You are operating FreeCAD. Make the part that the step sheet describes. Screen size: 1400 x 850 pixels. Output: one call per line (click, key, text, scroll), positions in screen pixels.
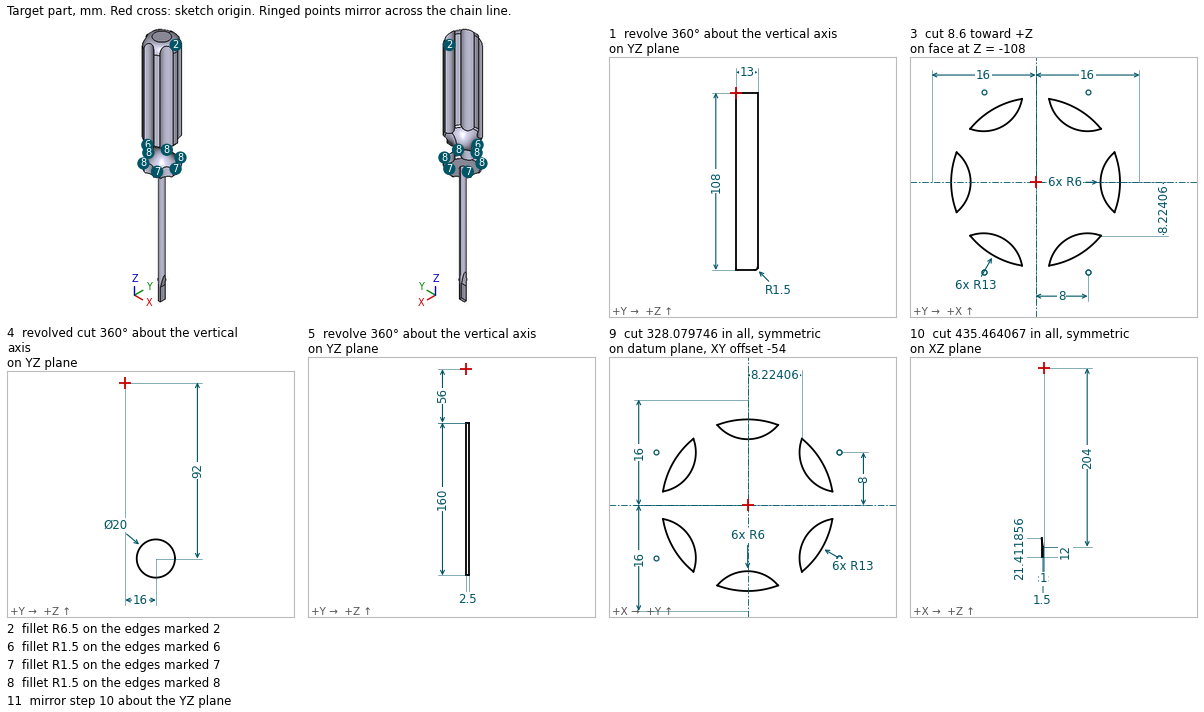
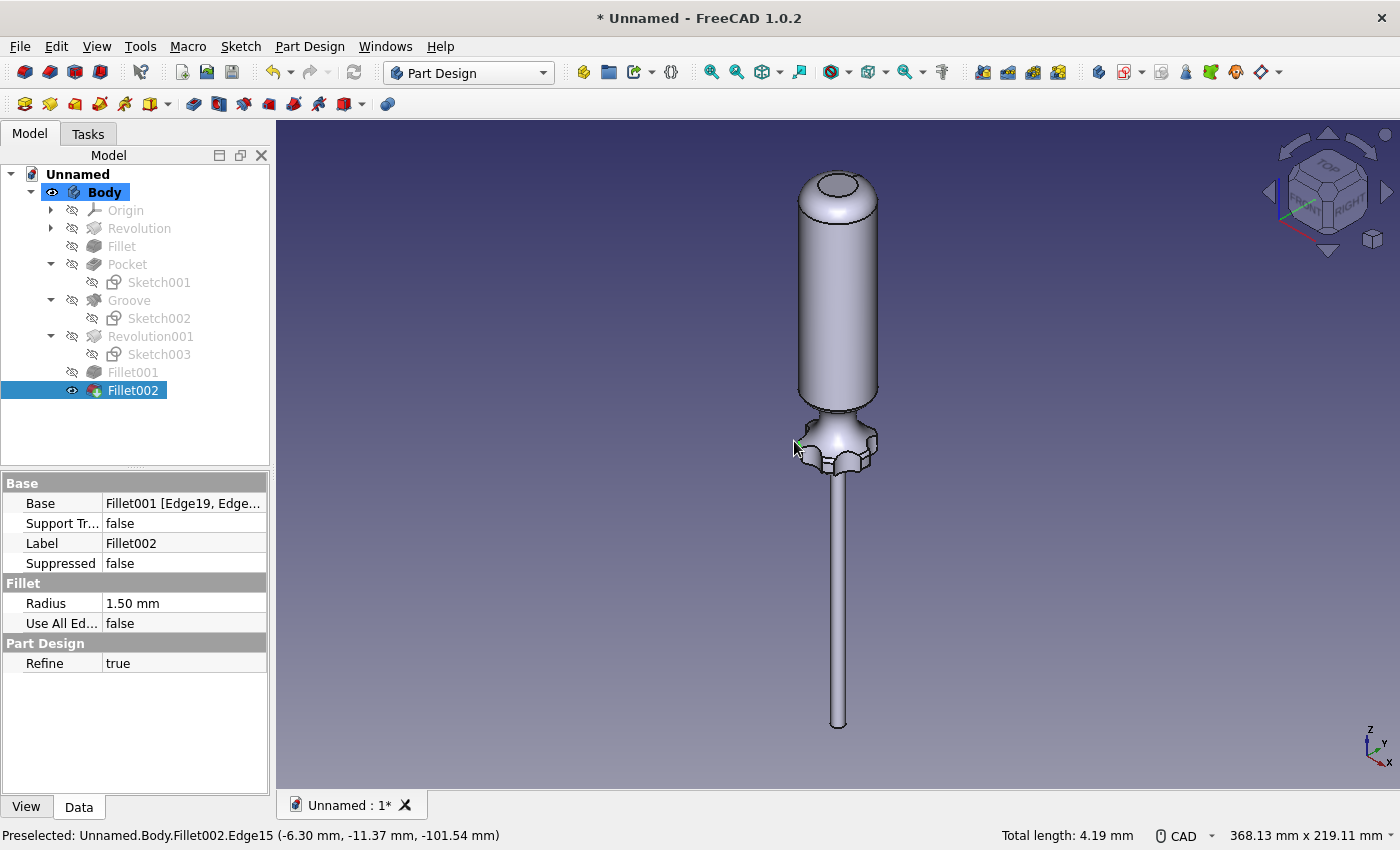
scroll(876, 431, up, 6)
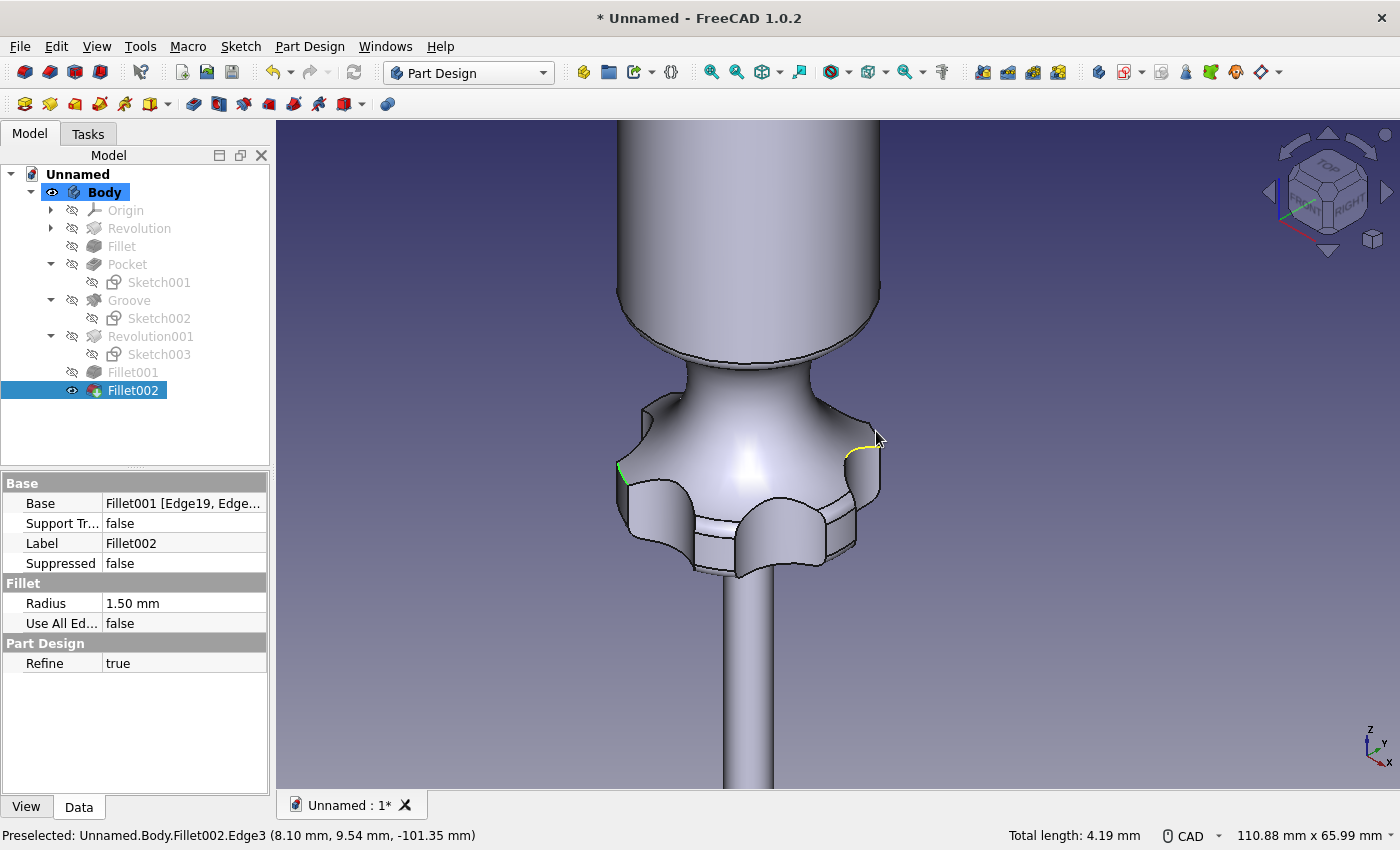
key(v)
key(f)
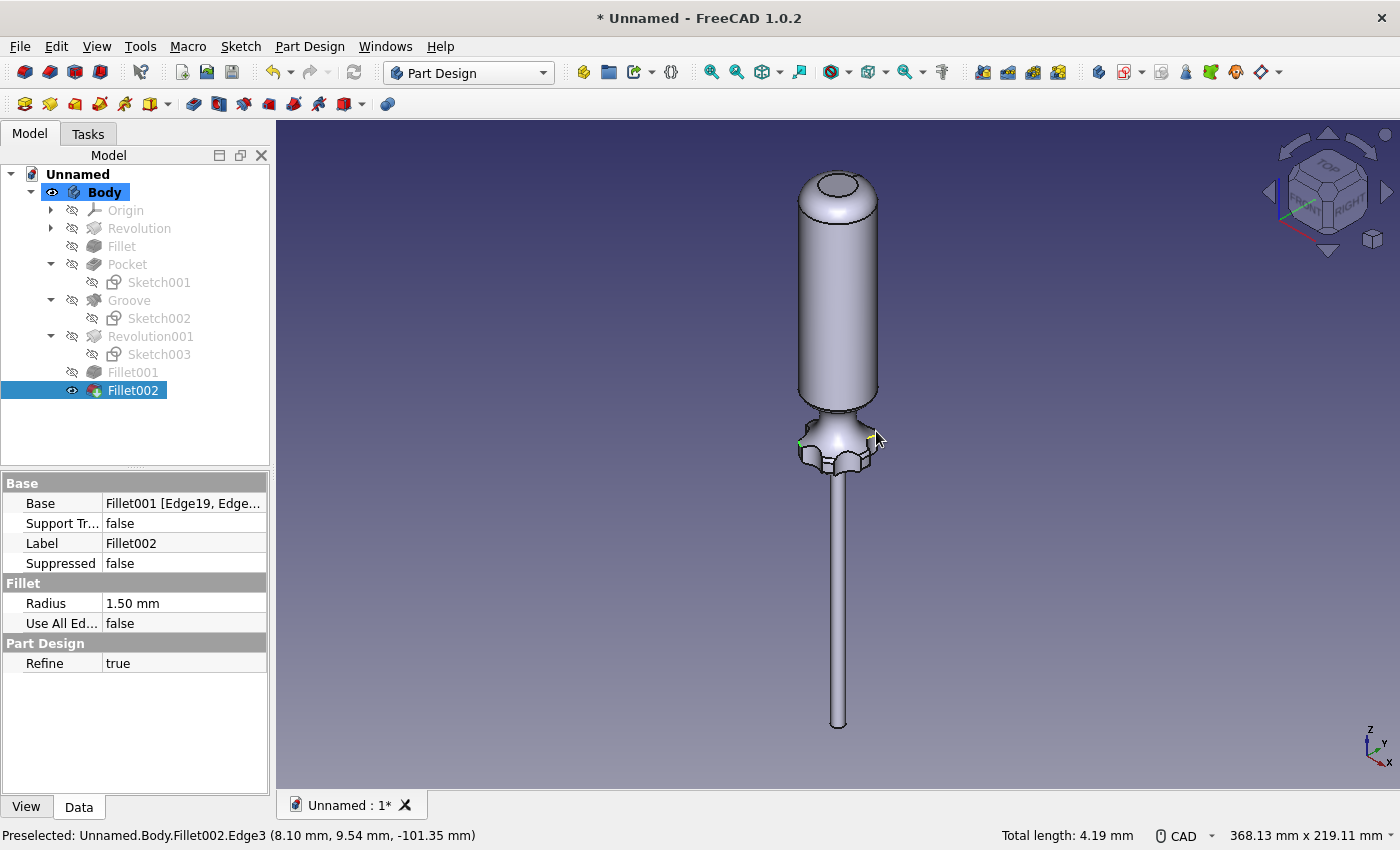
key(2)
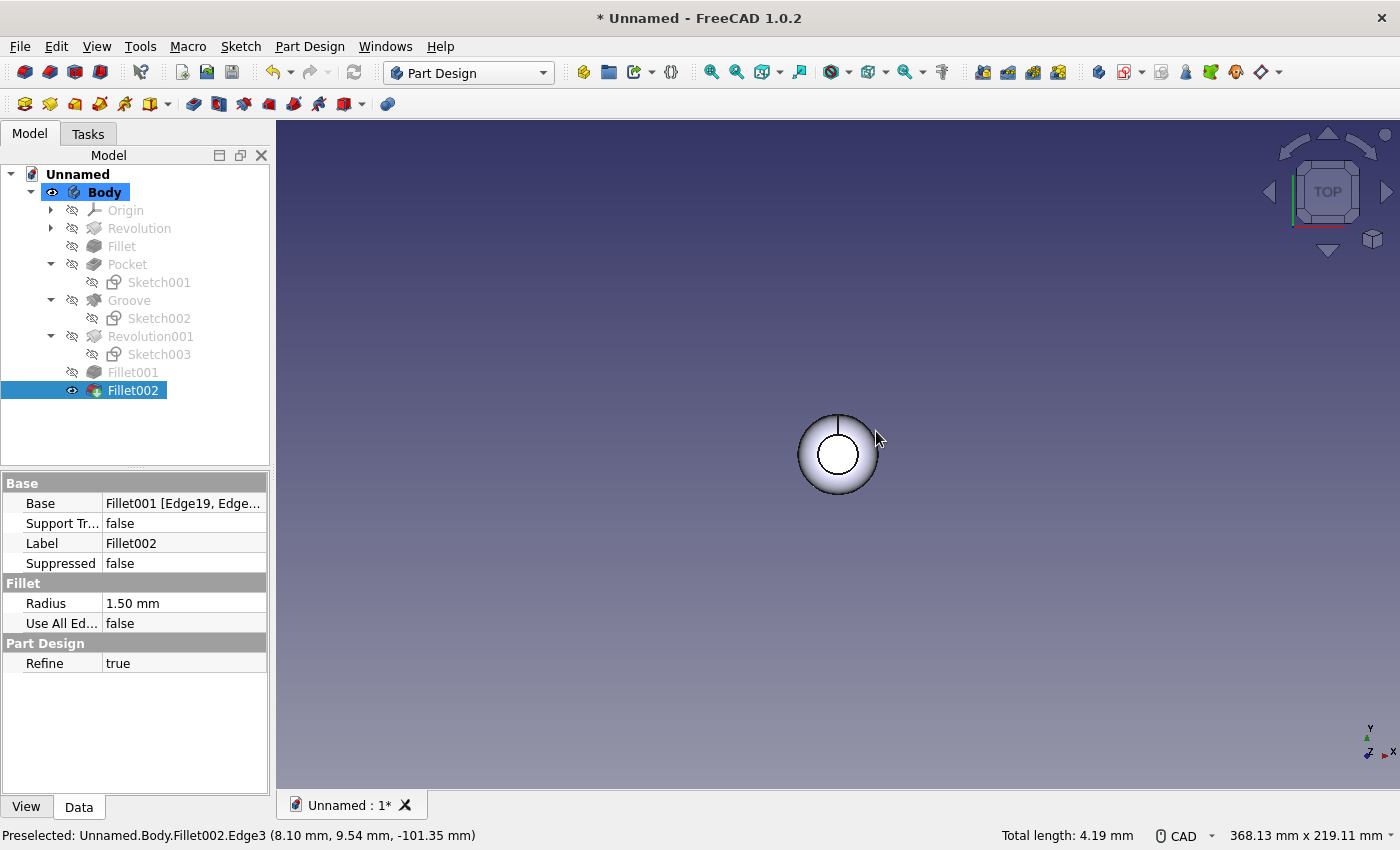
key(v)
key(f)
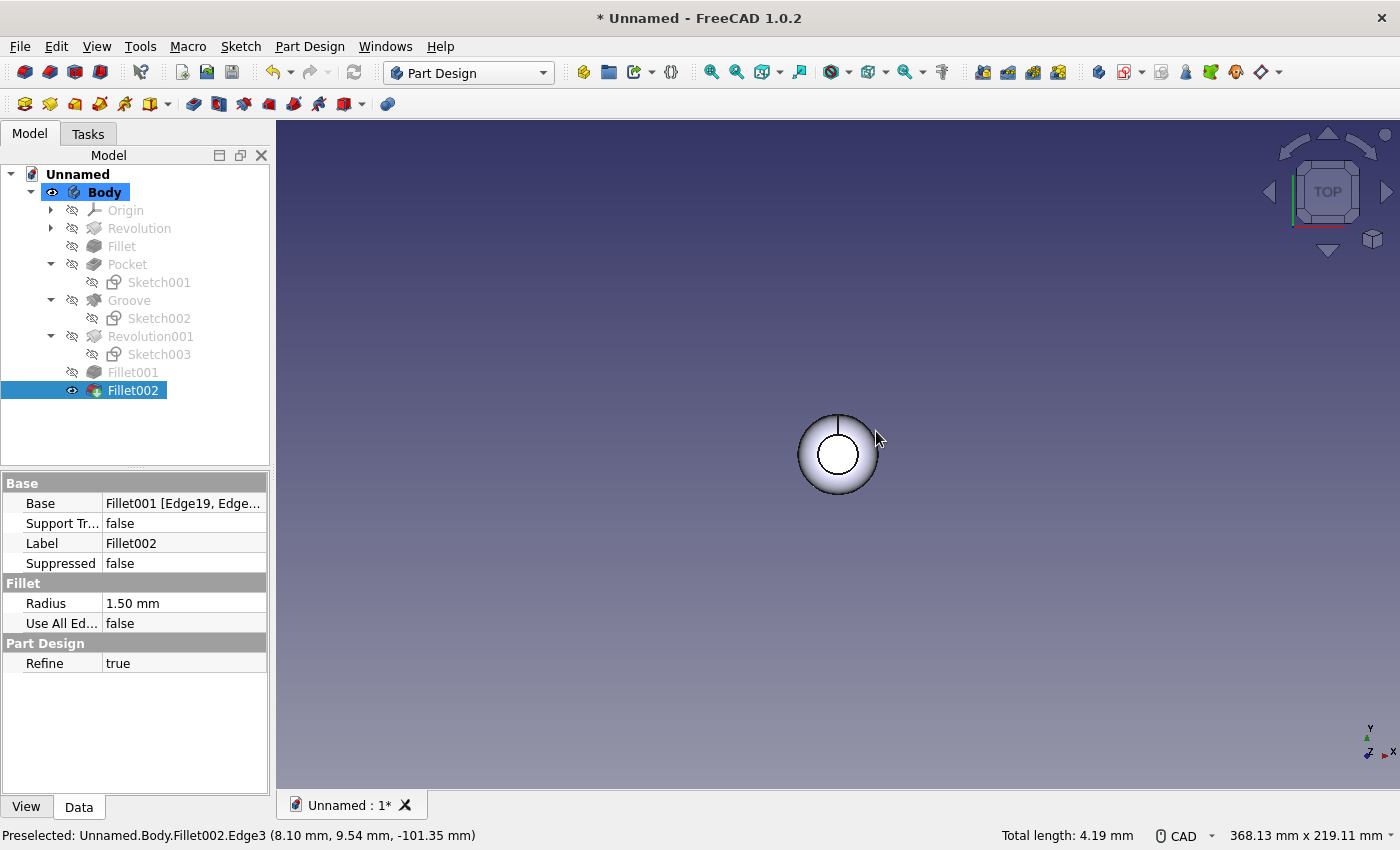
scroll(858, 419, up, 6)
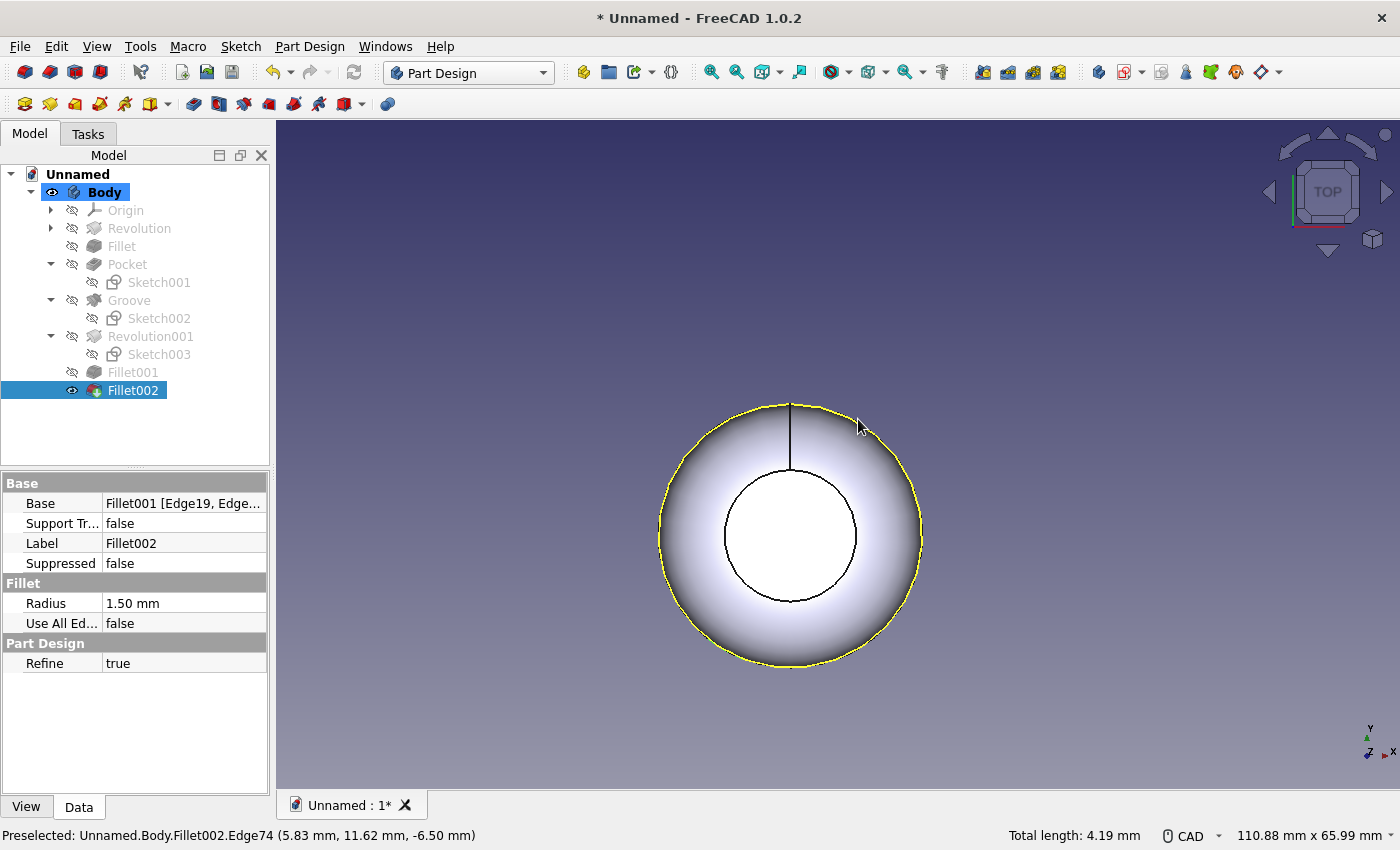
key(v)
key(f)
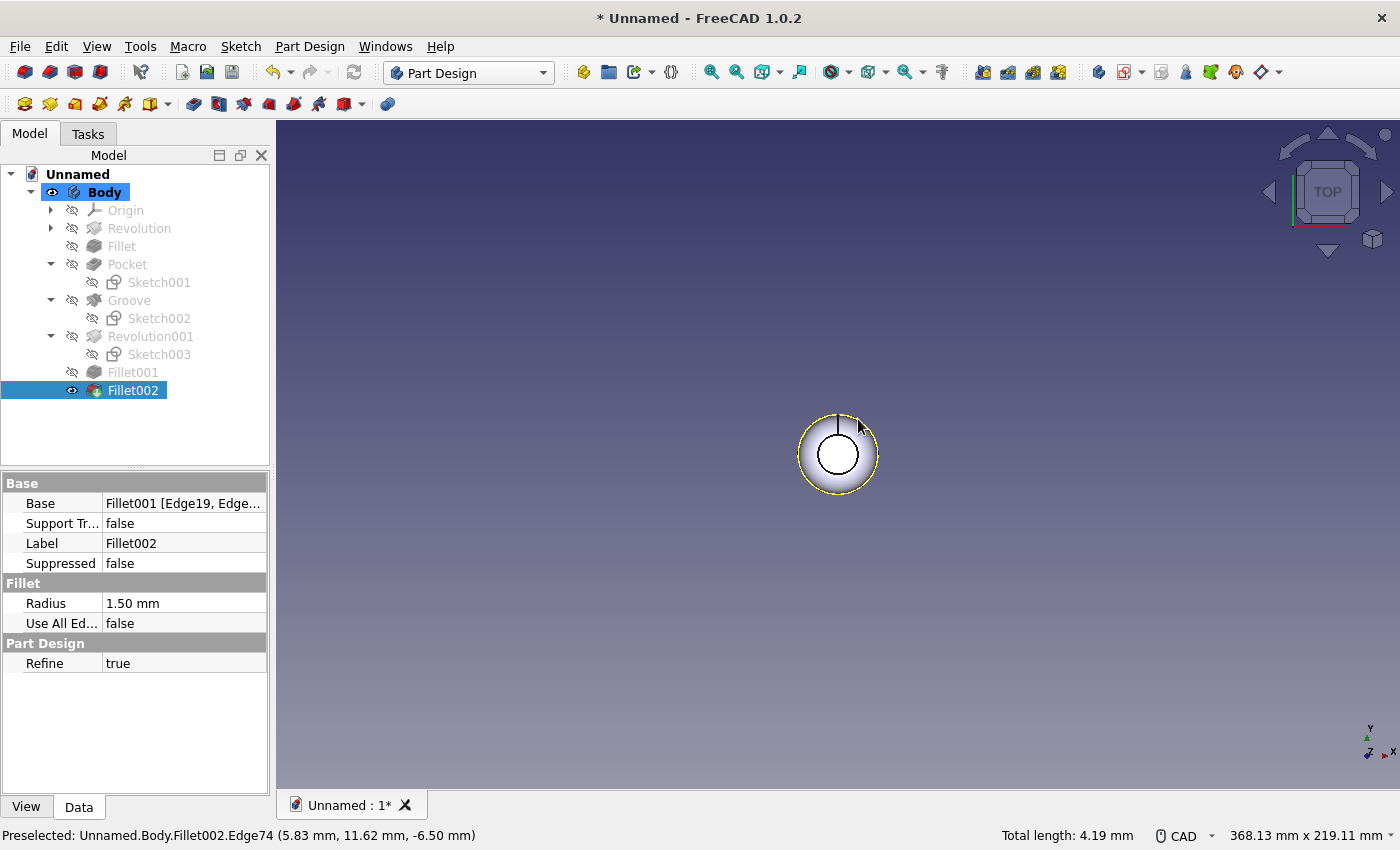
key(0)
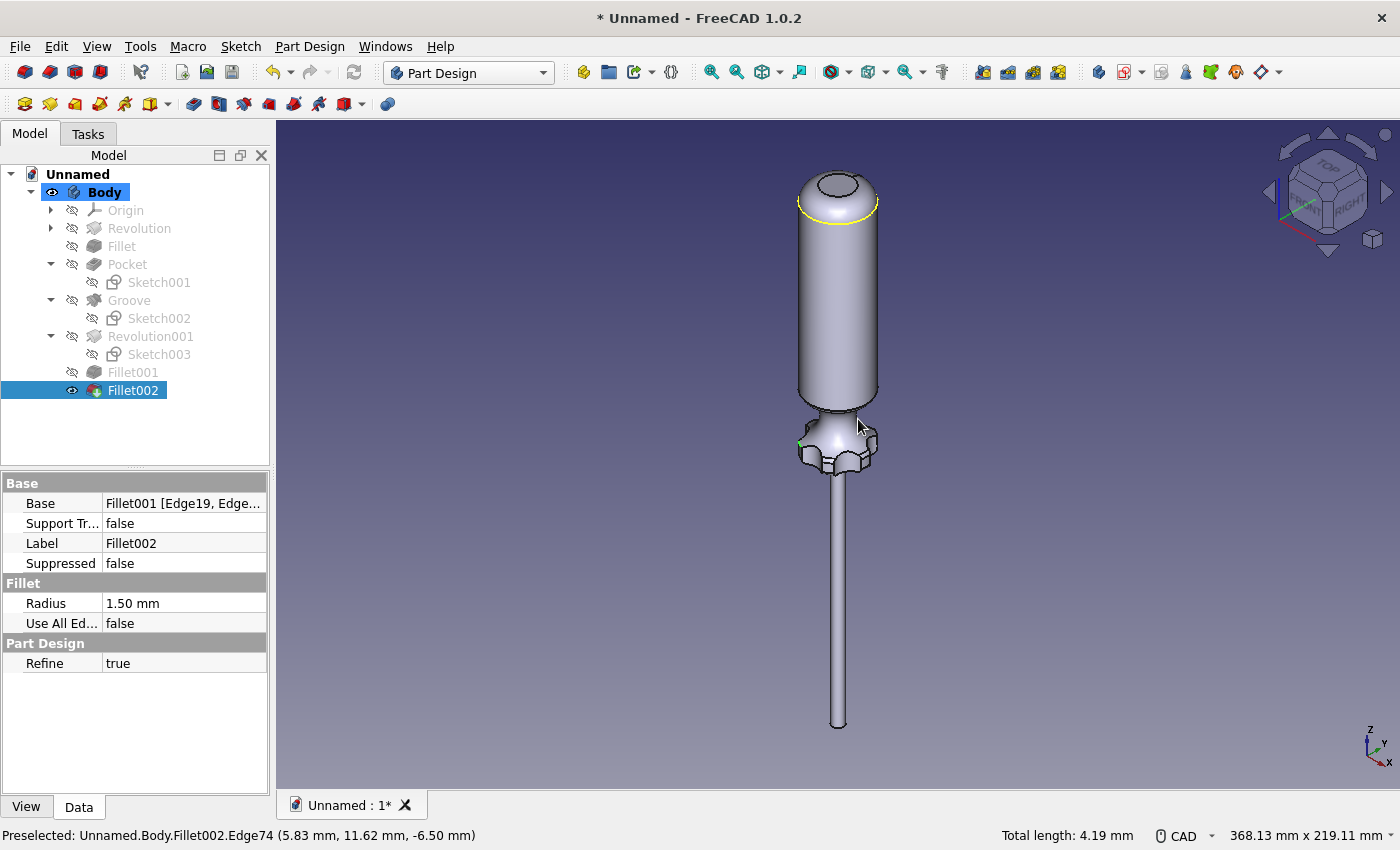
scroll(876, 431, up, 6)